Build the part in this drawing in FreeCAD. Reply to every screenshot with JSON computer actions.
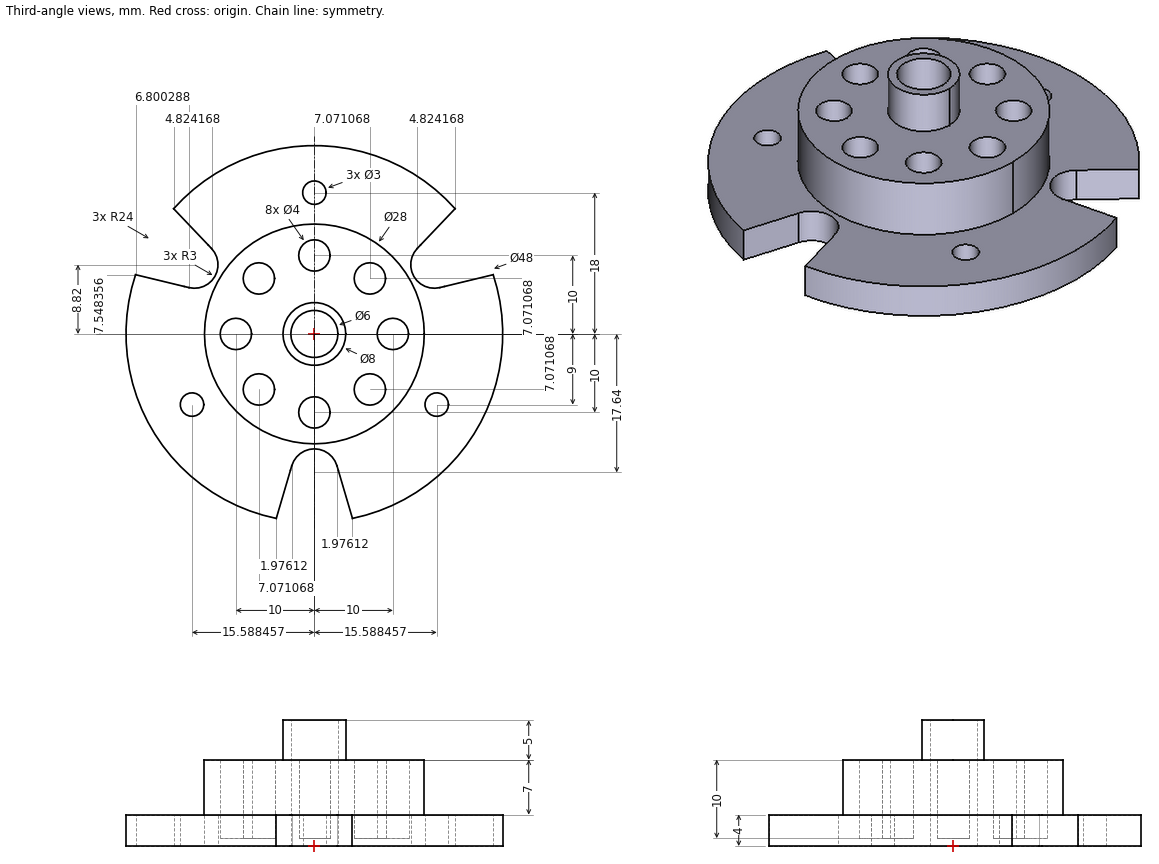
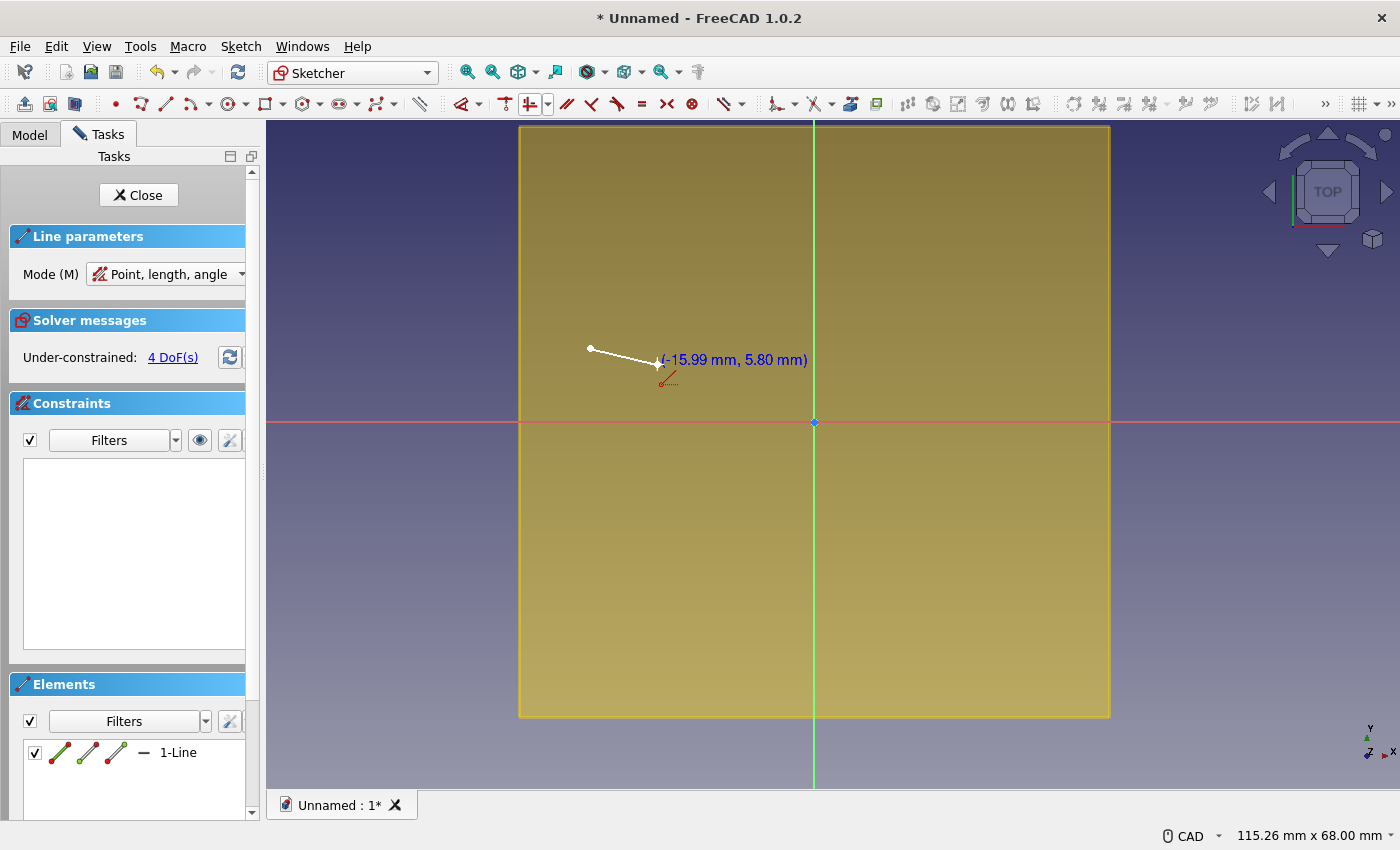
{"action": "left_click", "coordinate": [685, 315]}
{"action": "left_click", "coordinate": [638, 265]}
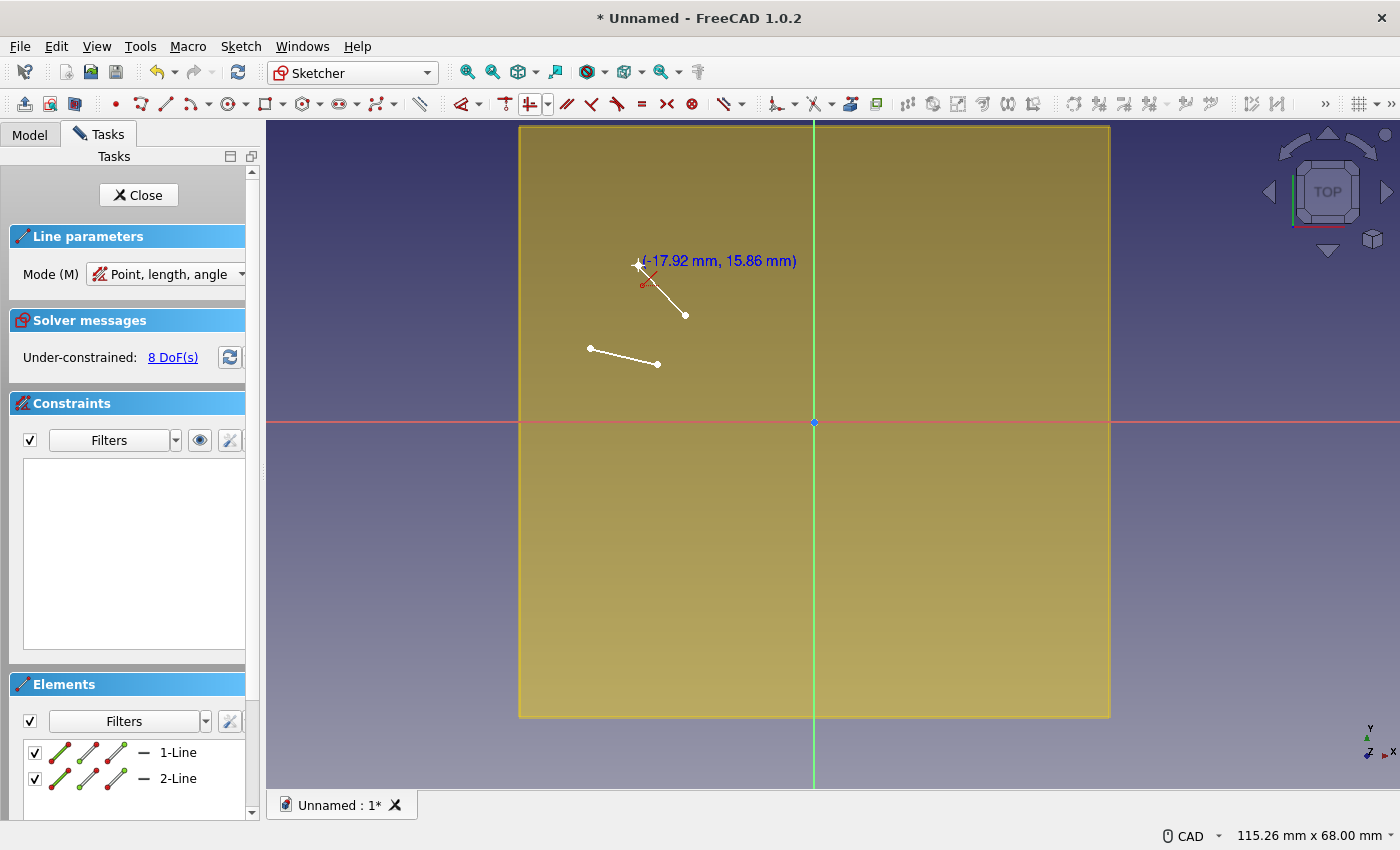
{"action": "left_click", "coordinate": [208, 104]}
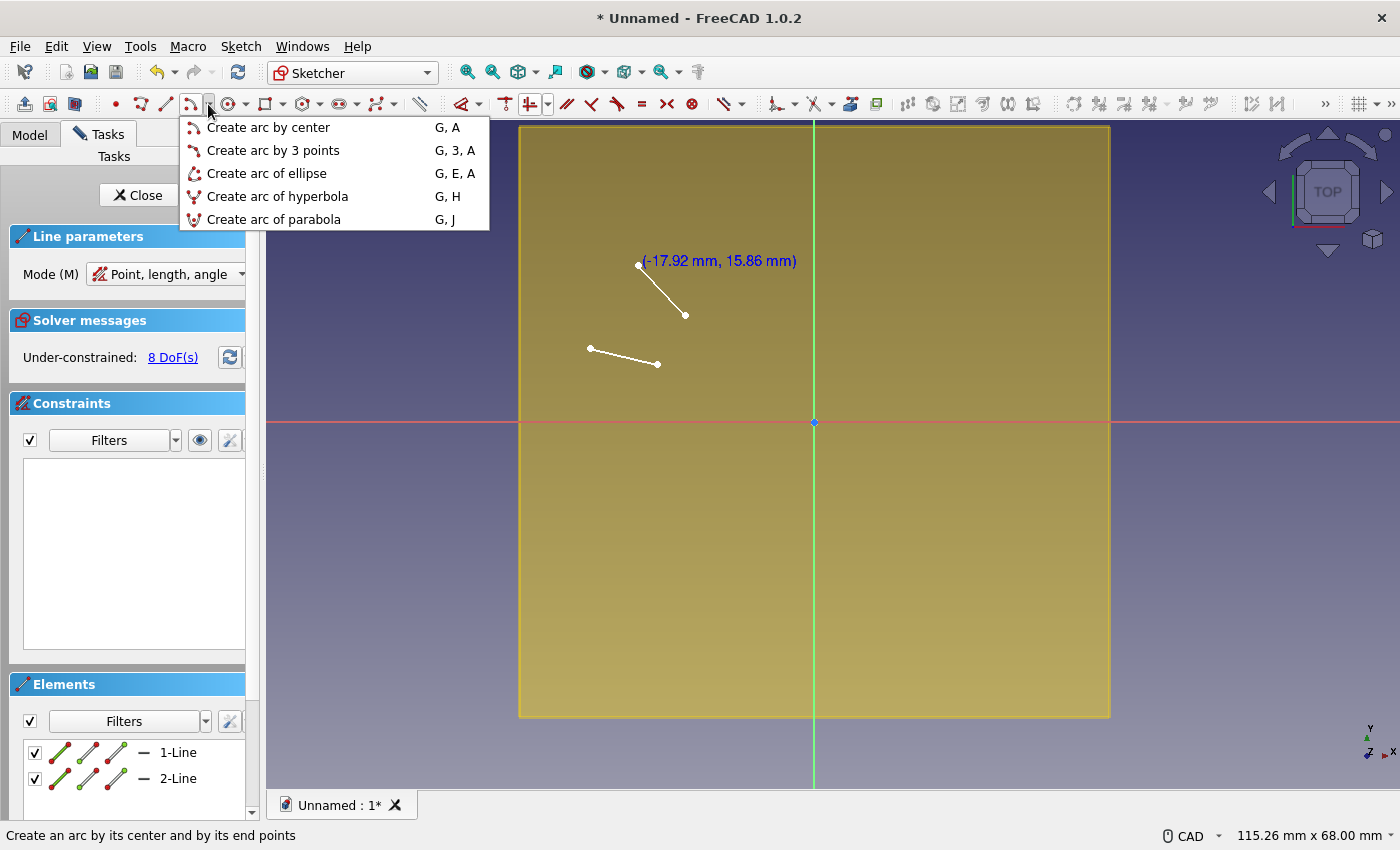
{"action": "left_click", "coordinate": [334, 150]}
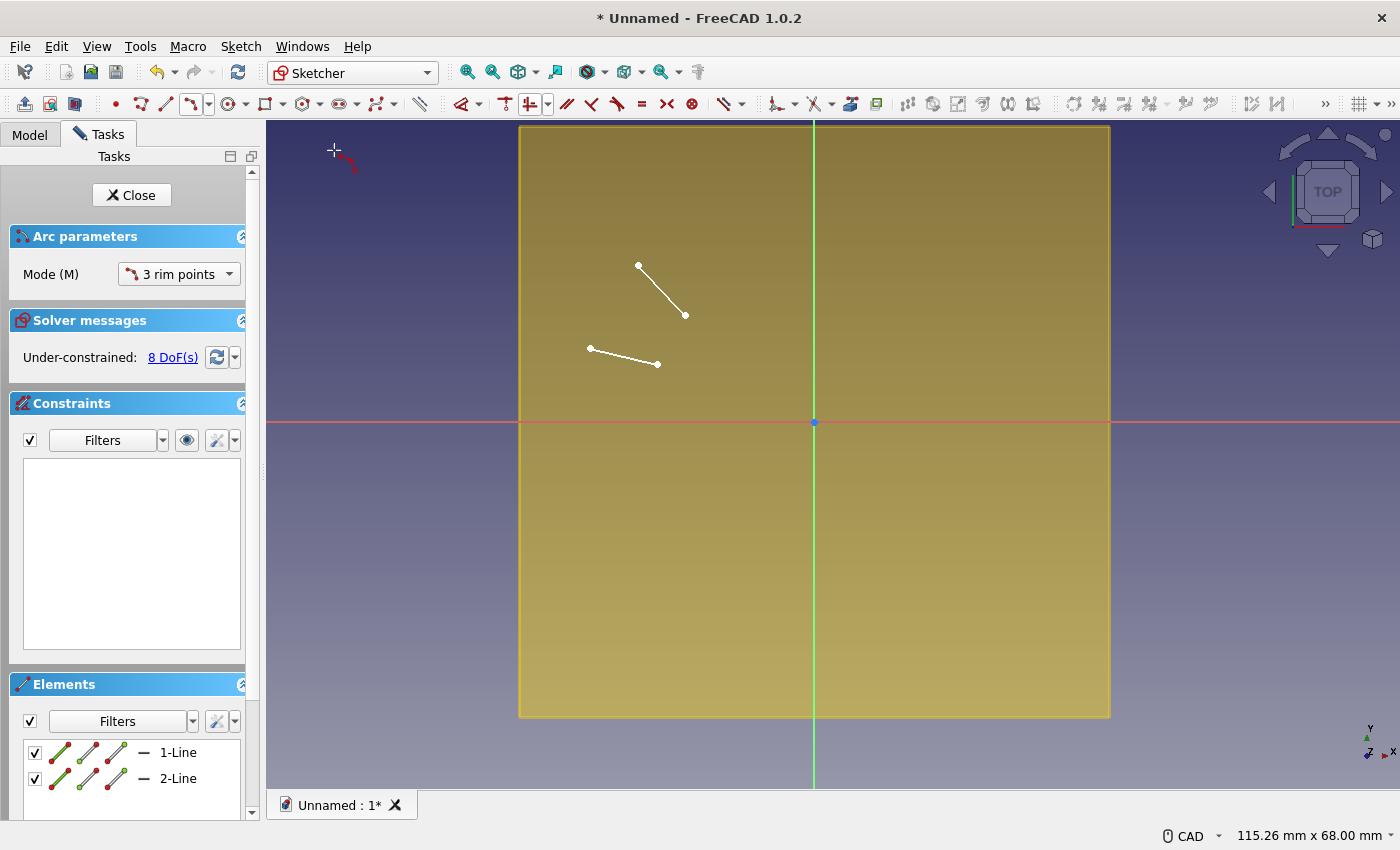
{"action": "left_click", "coordinate": [657, 365]}
{"action": "left_click", "coordinate": [685, 316]}
{"action": "left_click", "coordinate": [690, 350]}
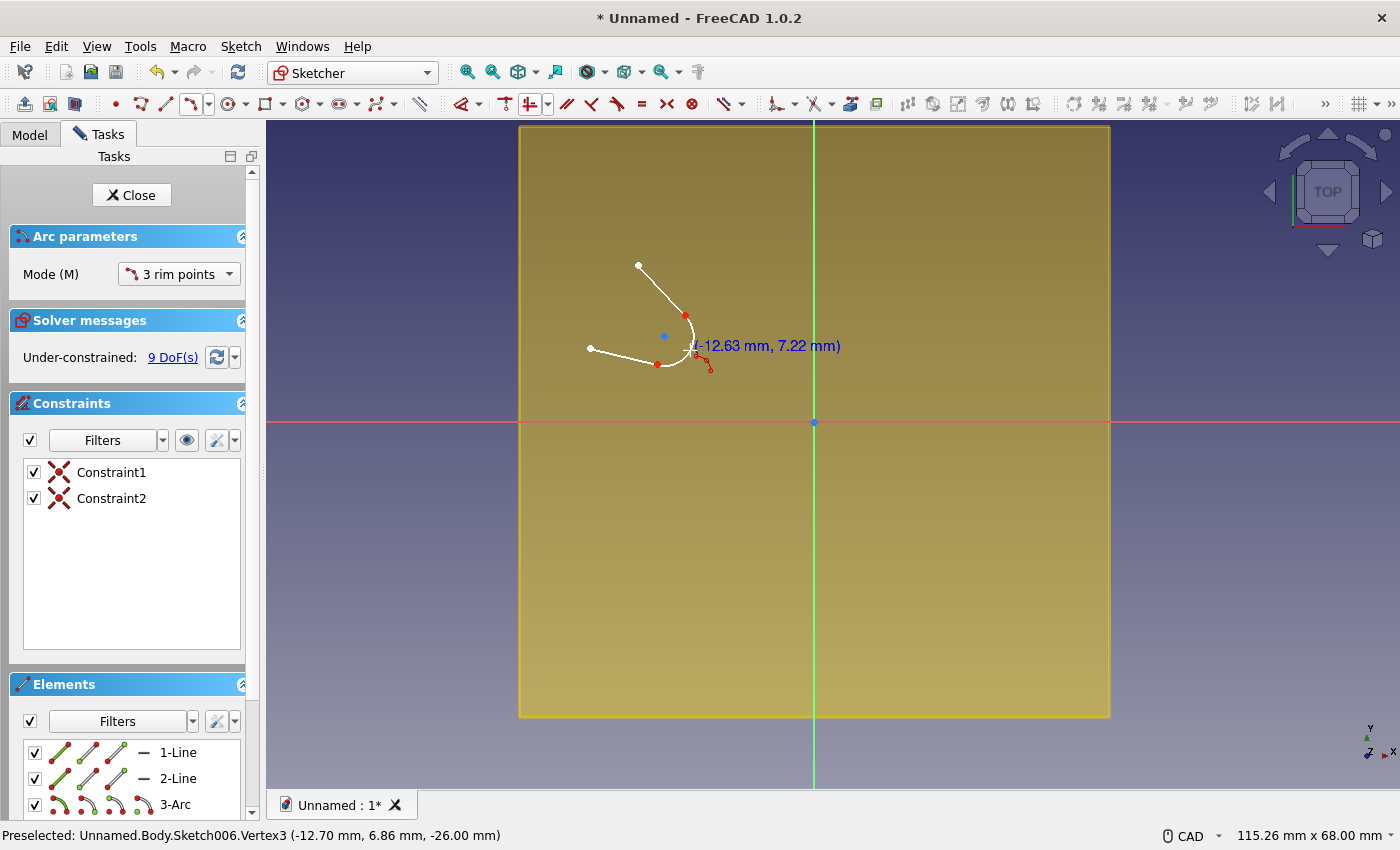
{"action": "left_click", "coordinate": [638, 266]}
{"action": "left_click", "coordinate": [590, 349]}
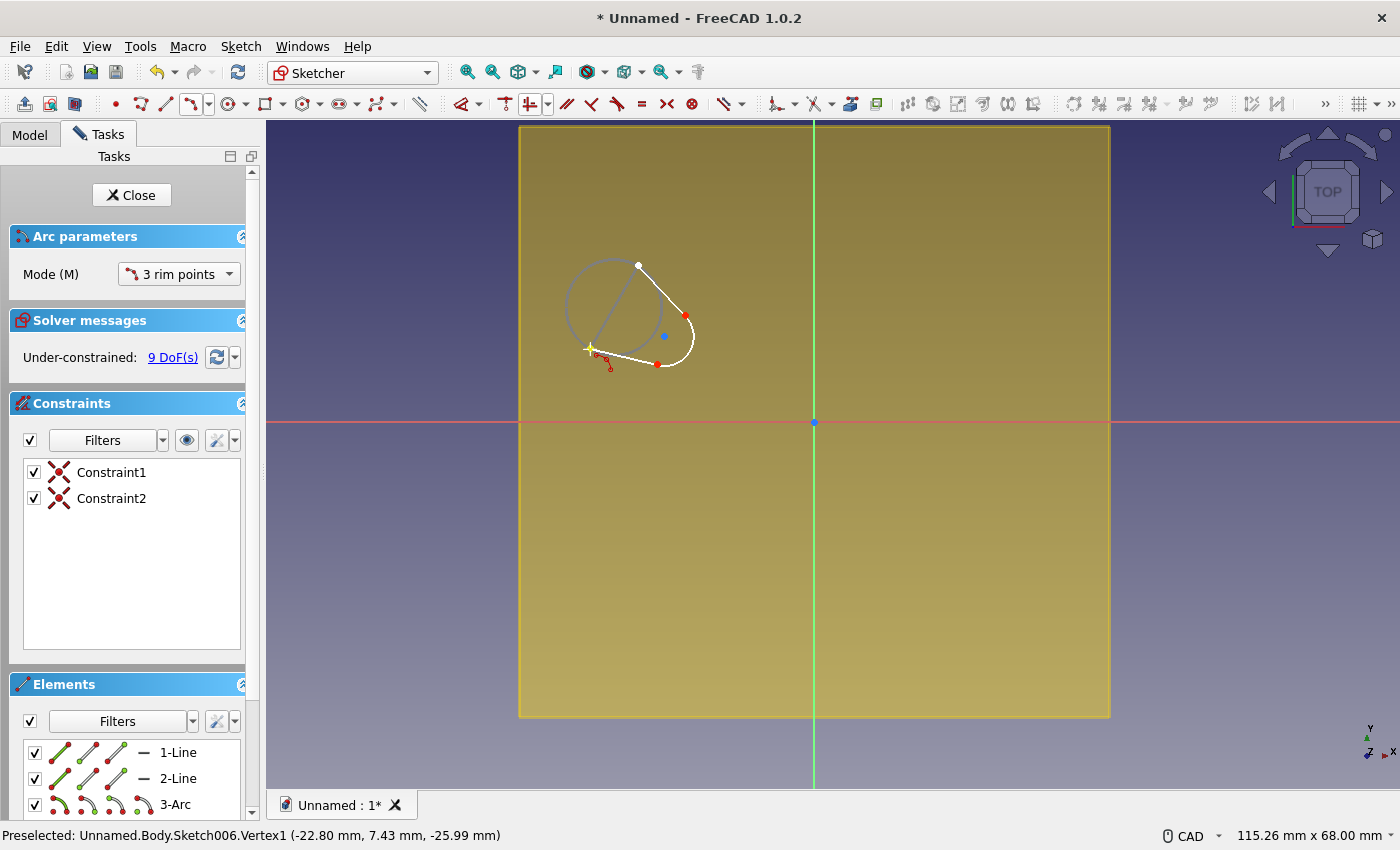
{"action": "scroll", "coordinate": [610, 304], "scroll_direction": "up", "scroll_amount": 6}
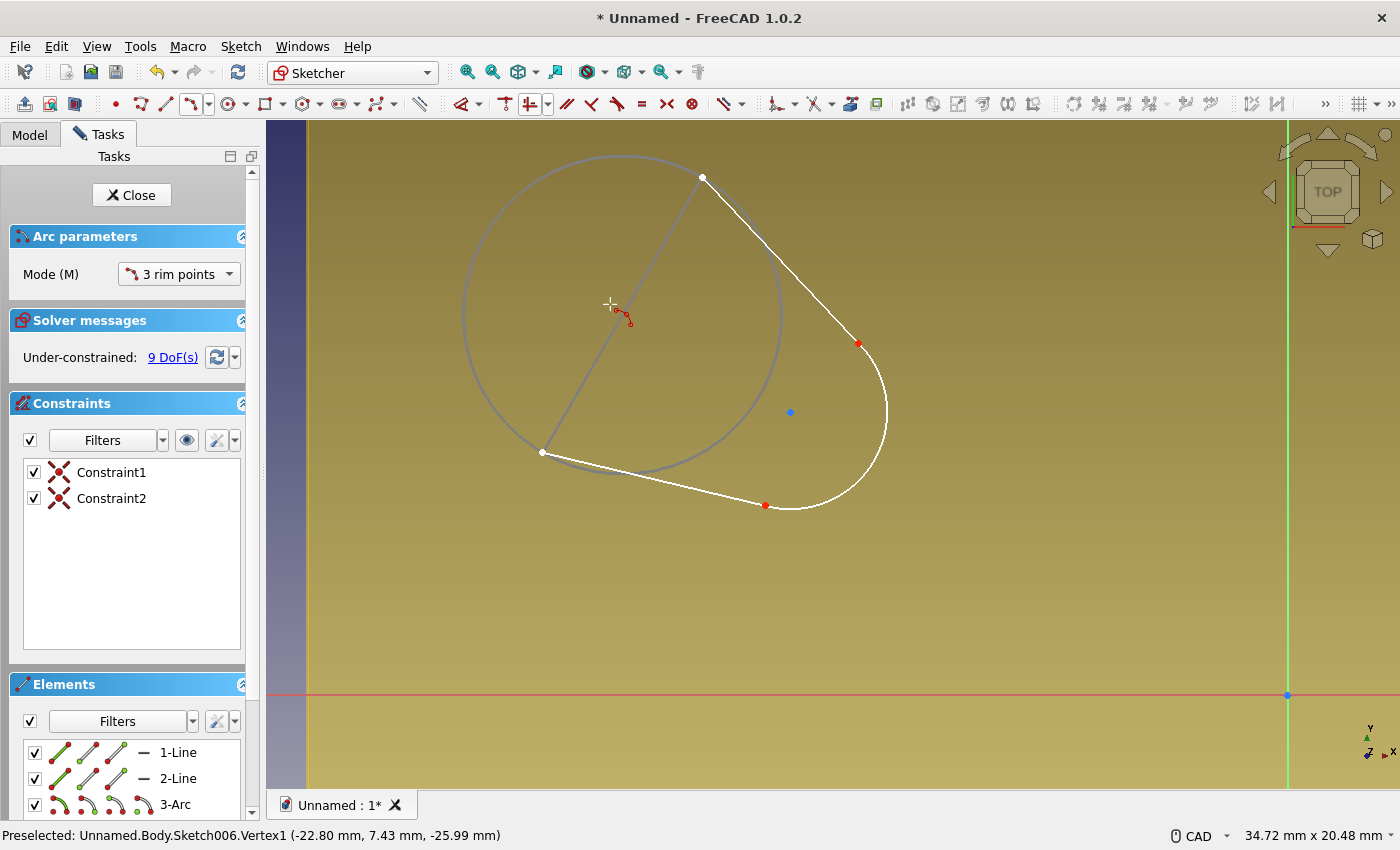
{"action": "left_click", "coordinate": [609, 303]}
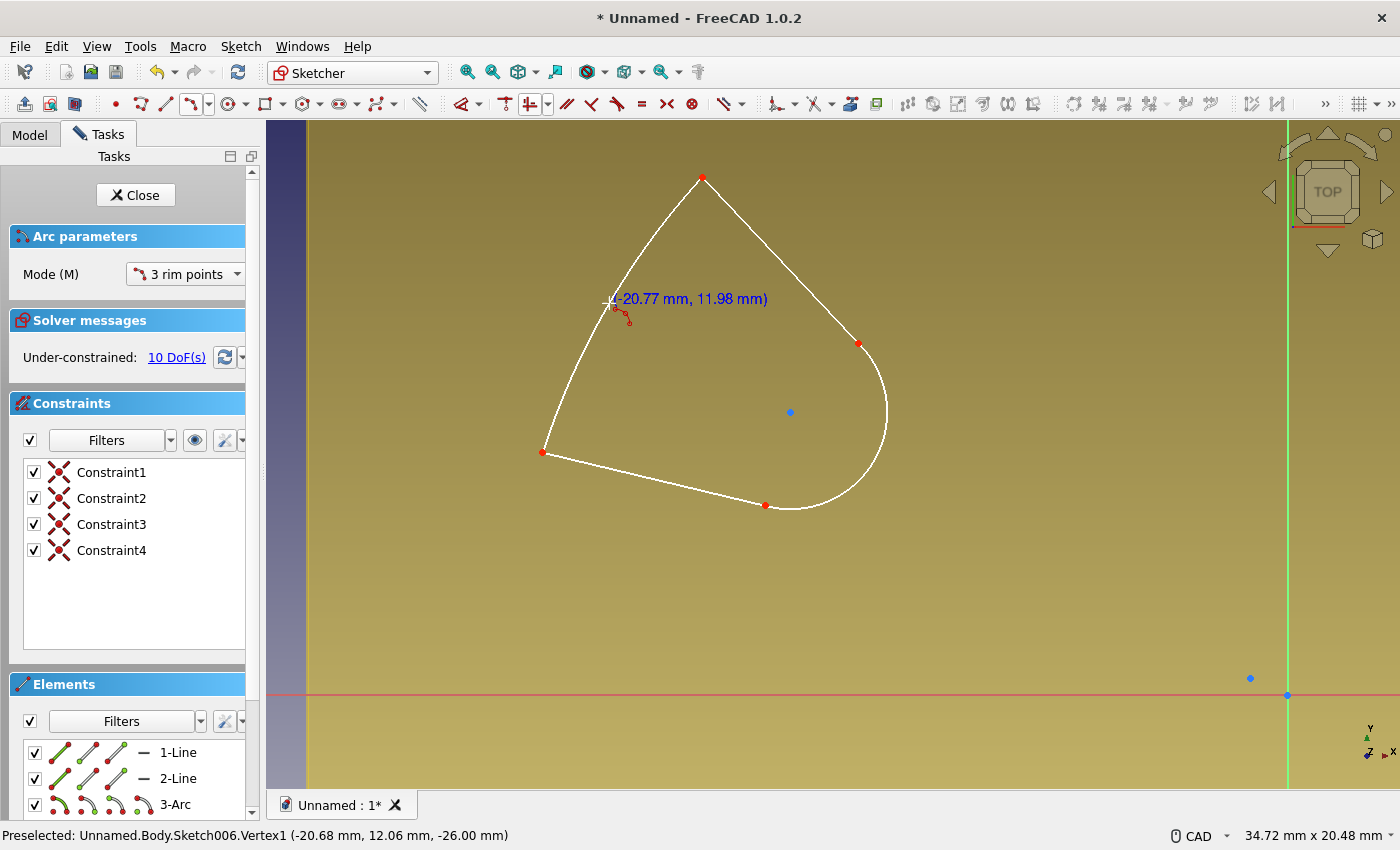
{"action": "key", "text": "g l"}